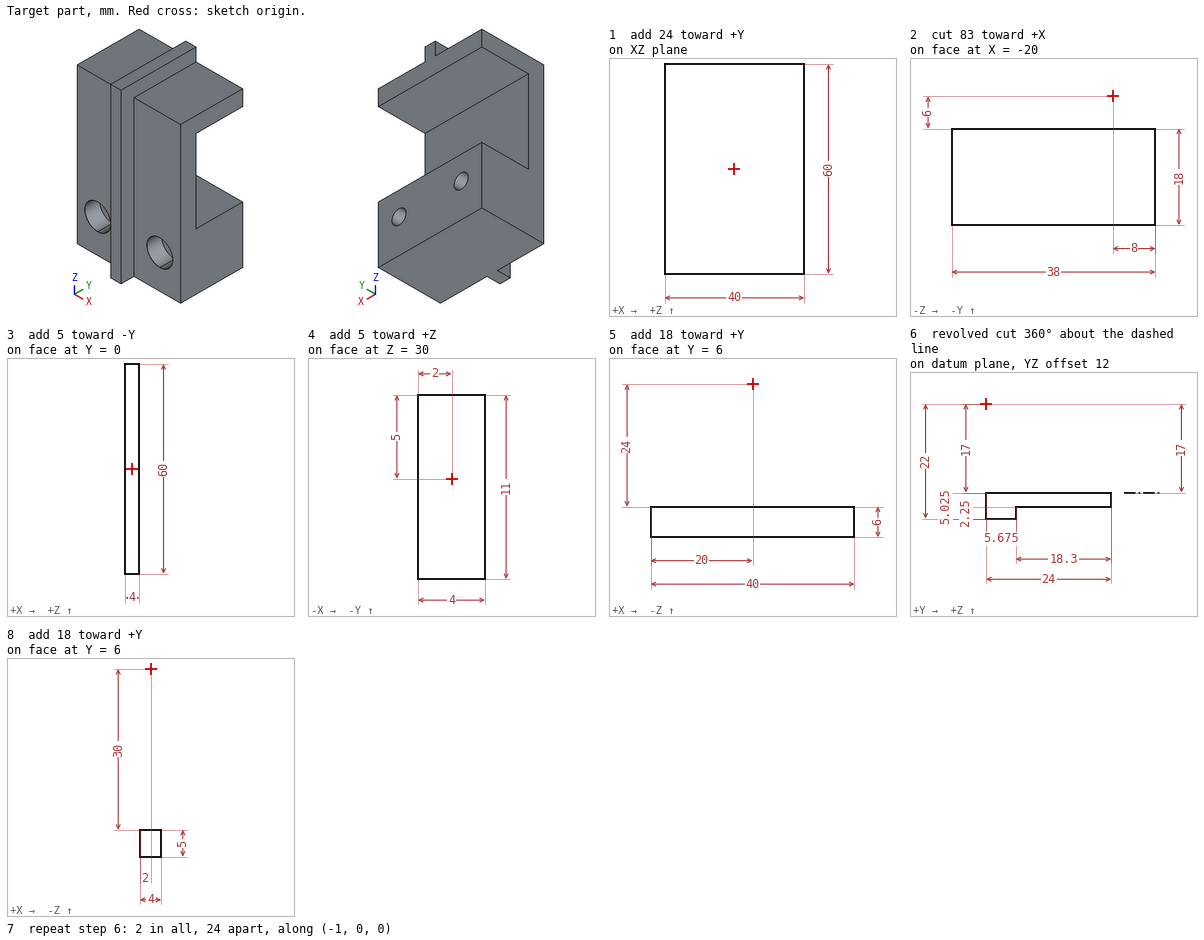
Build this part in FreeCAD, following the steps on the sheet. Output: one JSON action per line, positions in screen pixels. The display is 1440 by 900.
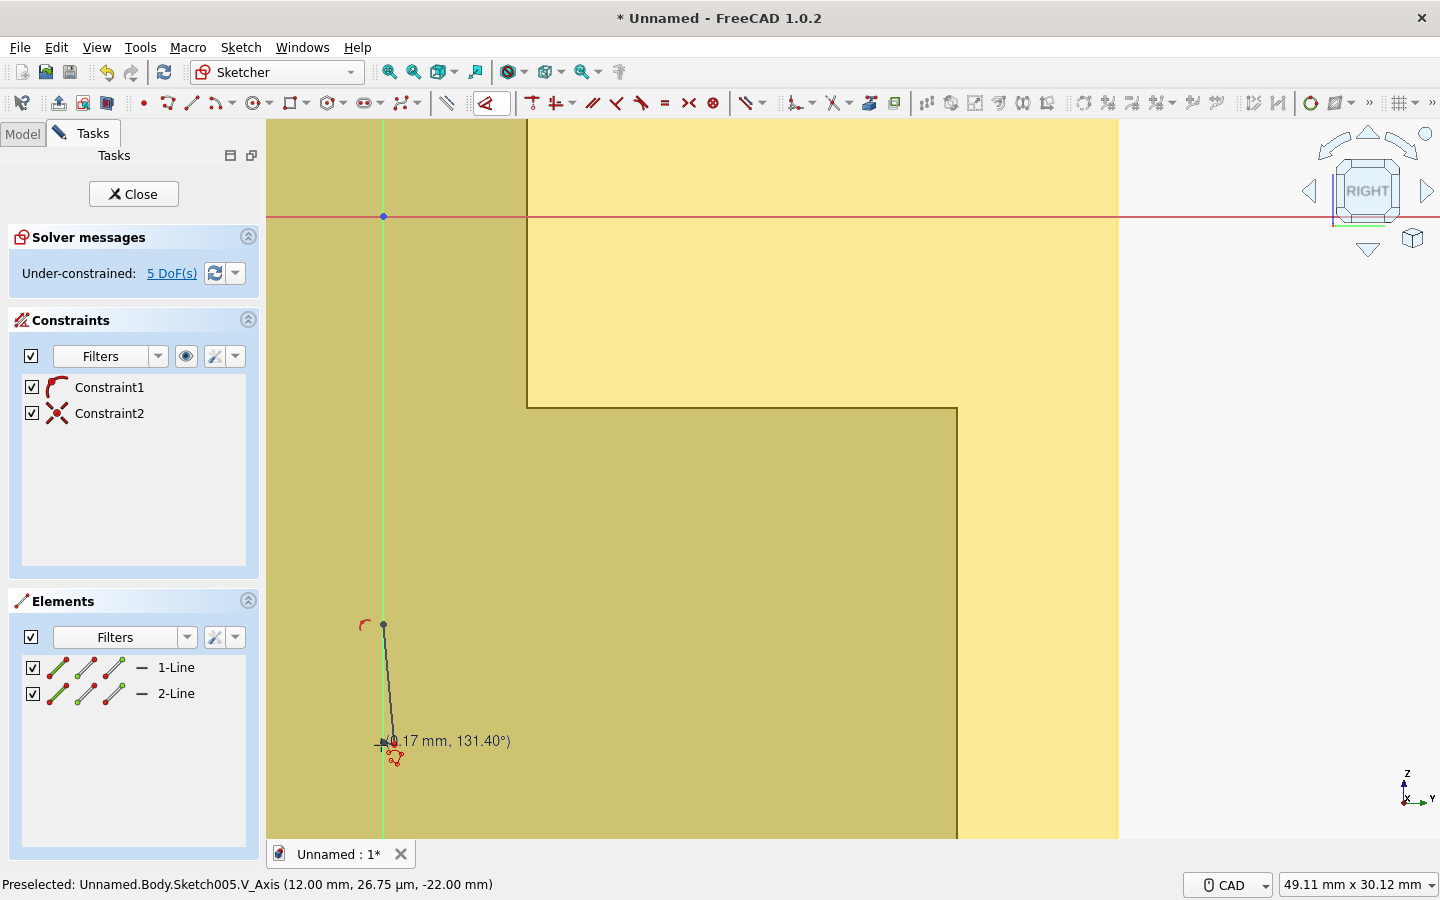
{"action": "left_click", "coordinate": [519, 743]}
{"action": "left_click", "coordinate": [519, 689]}
{"action": "left_click", "coordinate": [957, 689]}
{"action": "left_click", "coordinate": [957, 623]}
{"action": "left_click", "coordinate": [383, 625]}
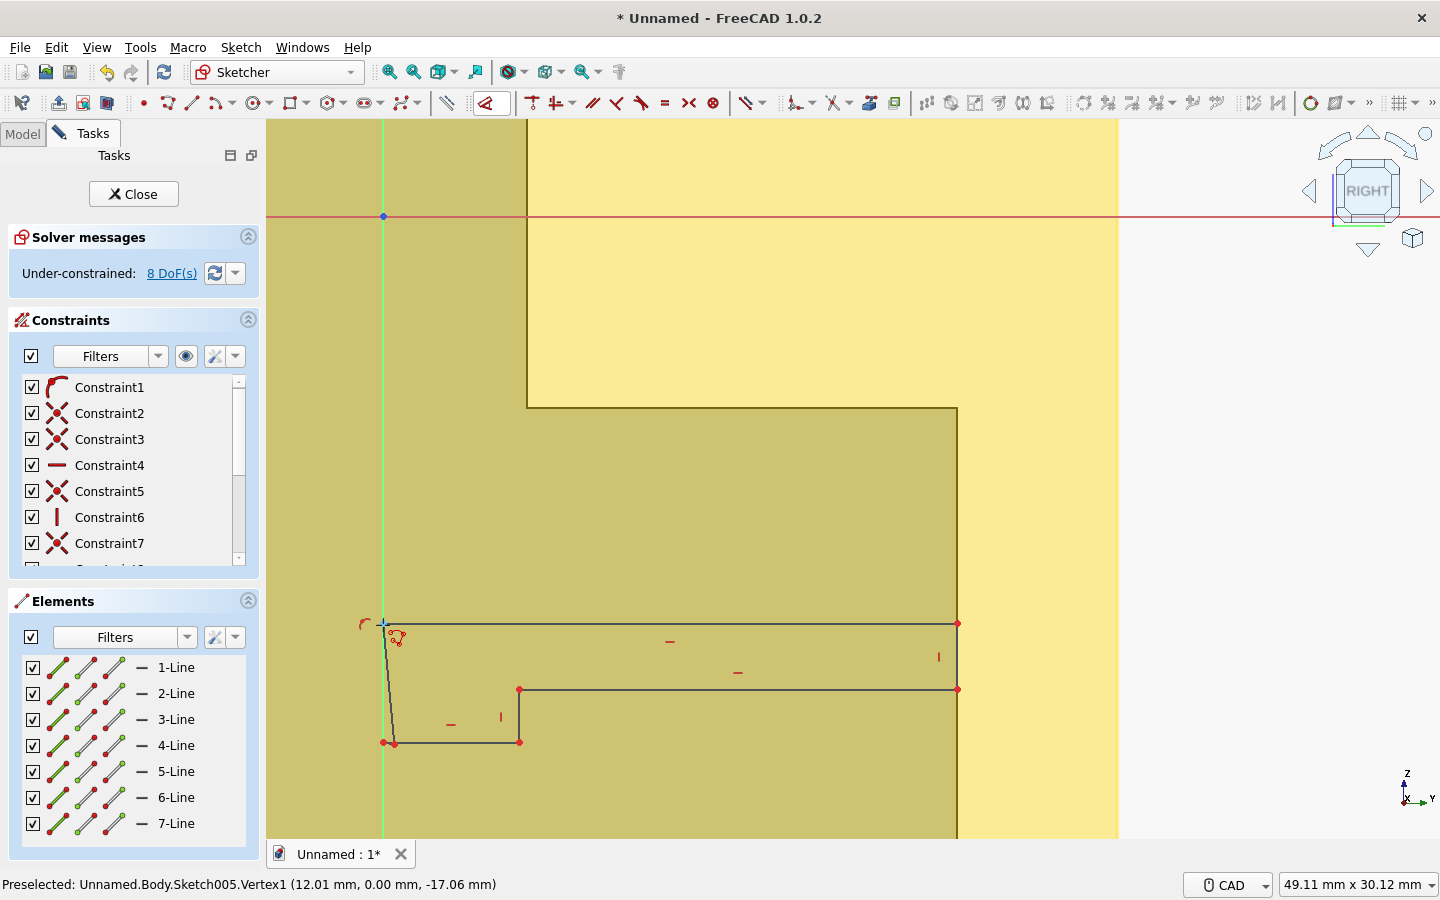
{"action": "key", "text": "g l"}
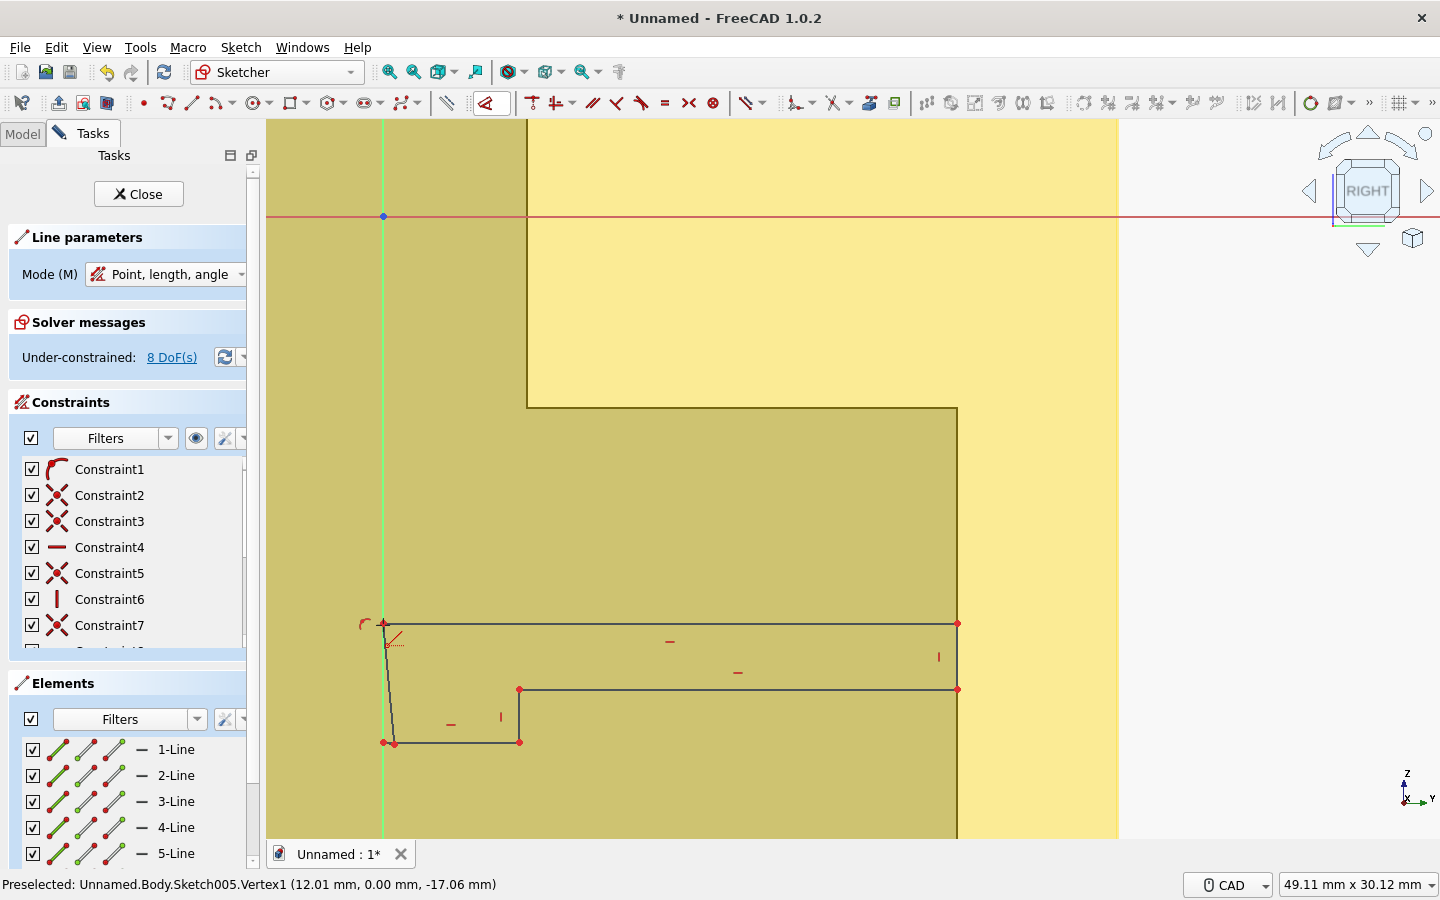
{"action": "left_click", "coordinate": [1014, 623]}
{"action": "left_click", "coordinate": [1186, 623]}
{"action": "key", "text": "Escape"}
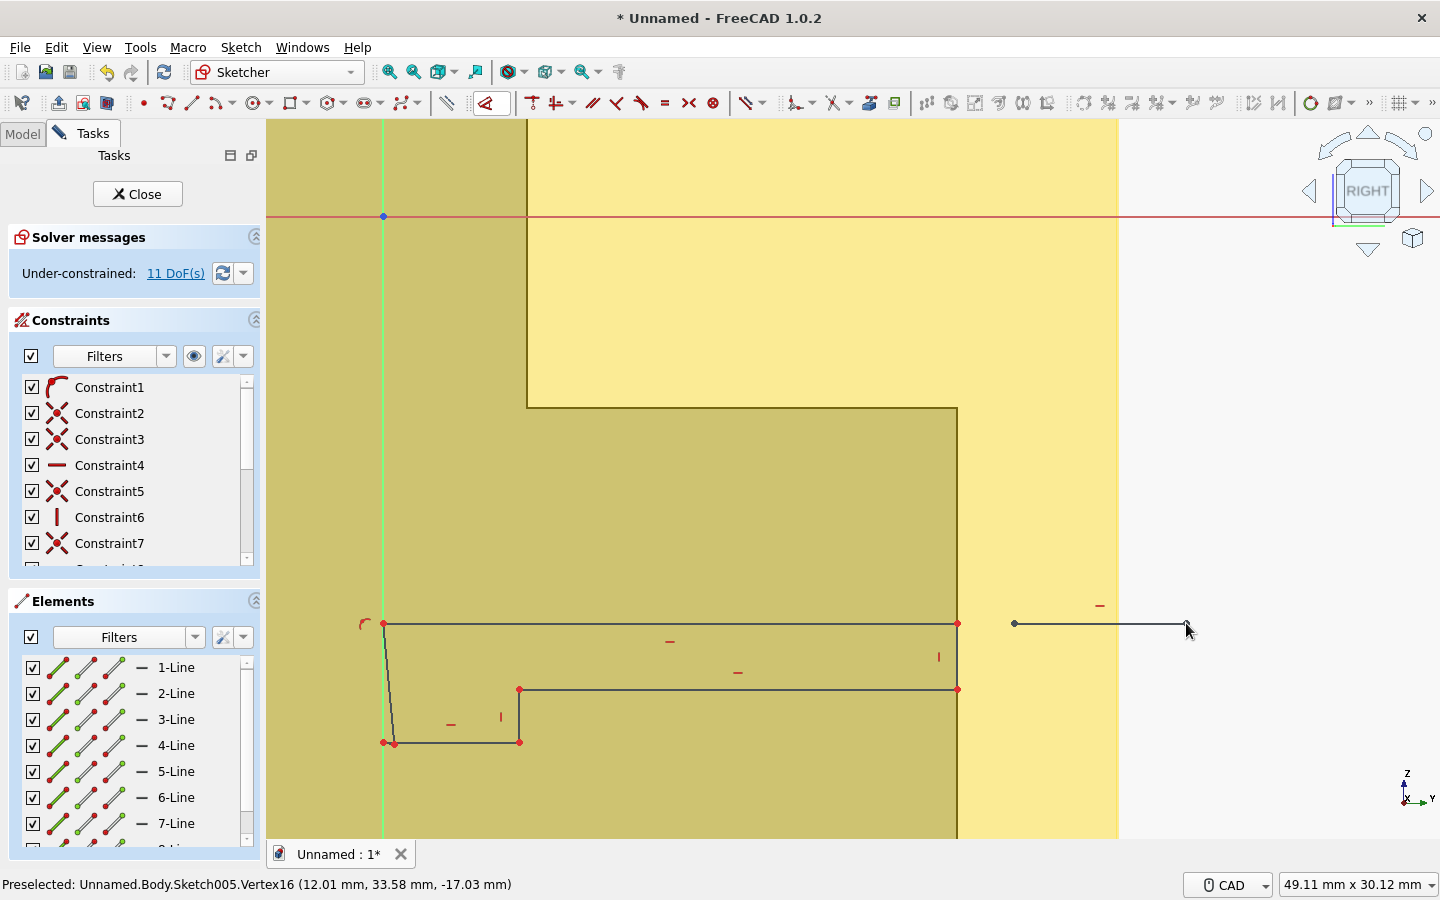
{"action": "left_click", "coordinate": [1066, 624]}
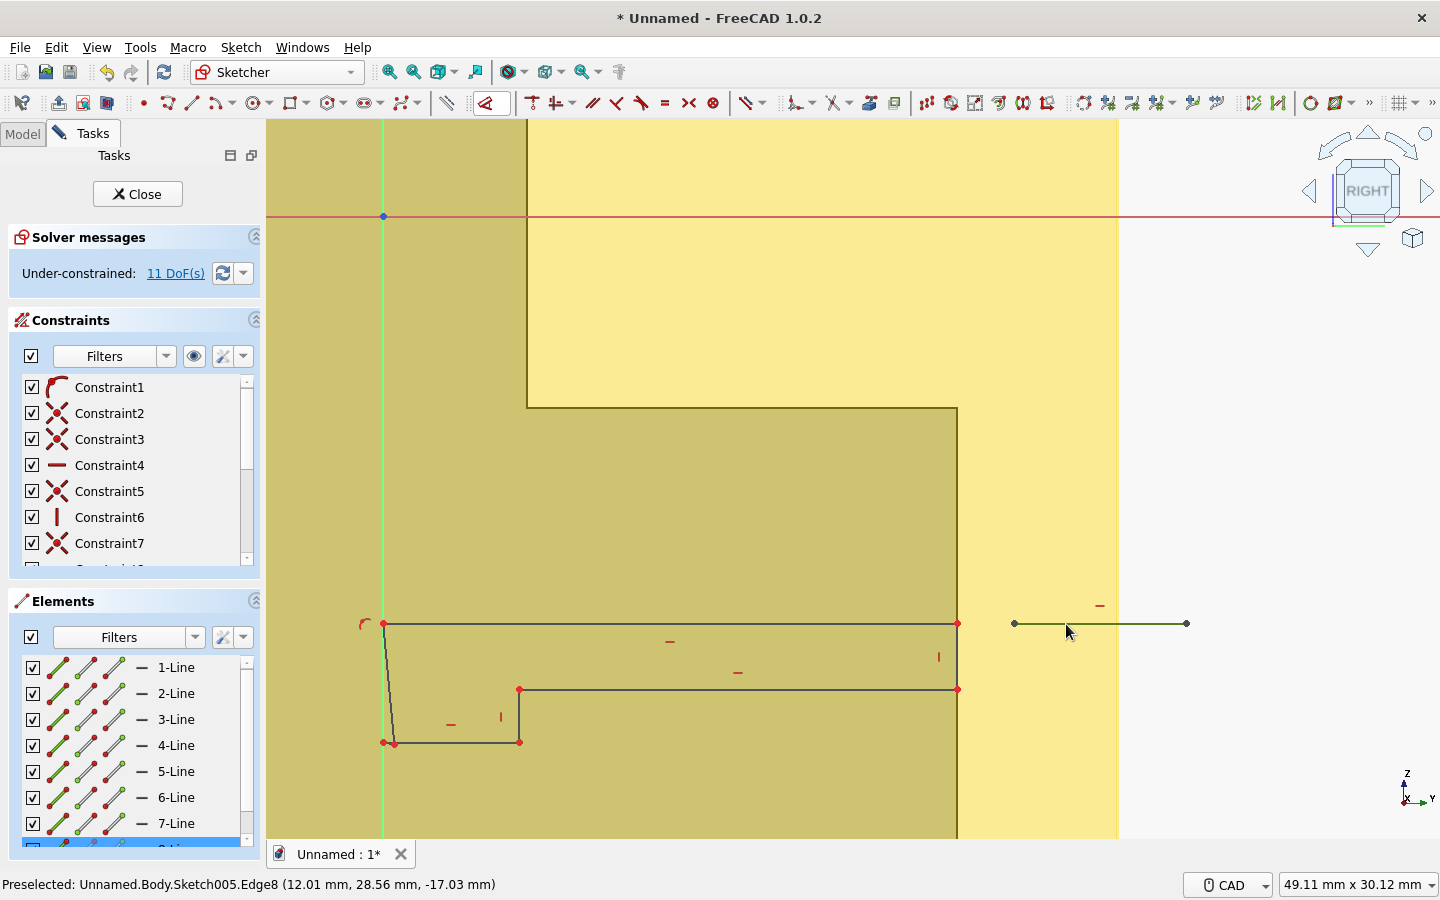
{"action": "key", "text": "g n"}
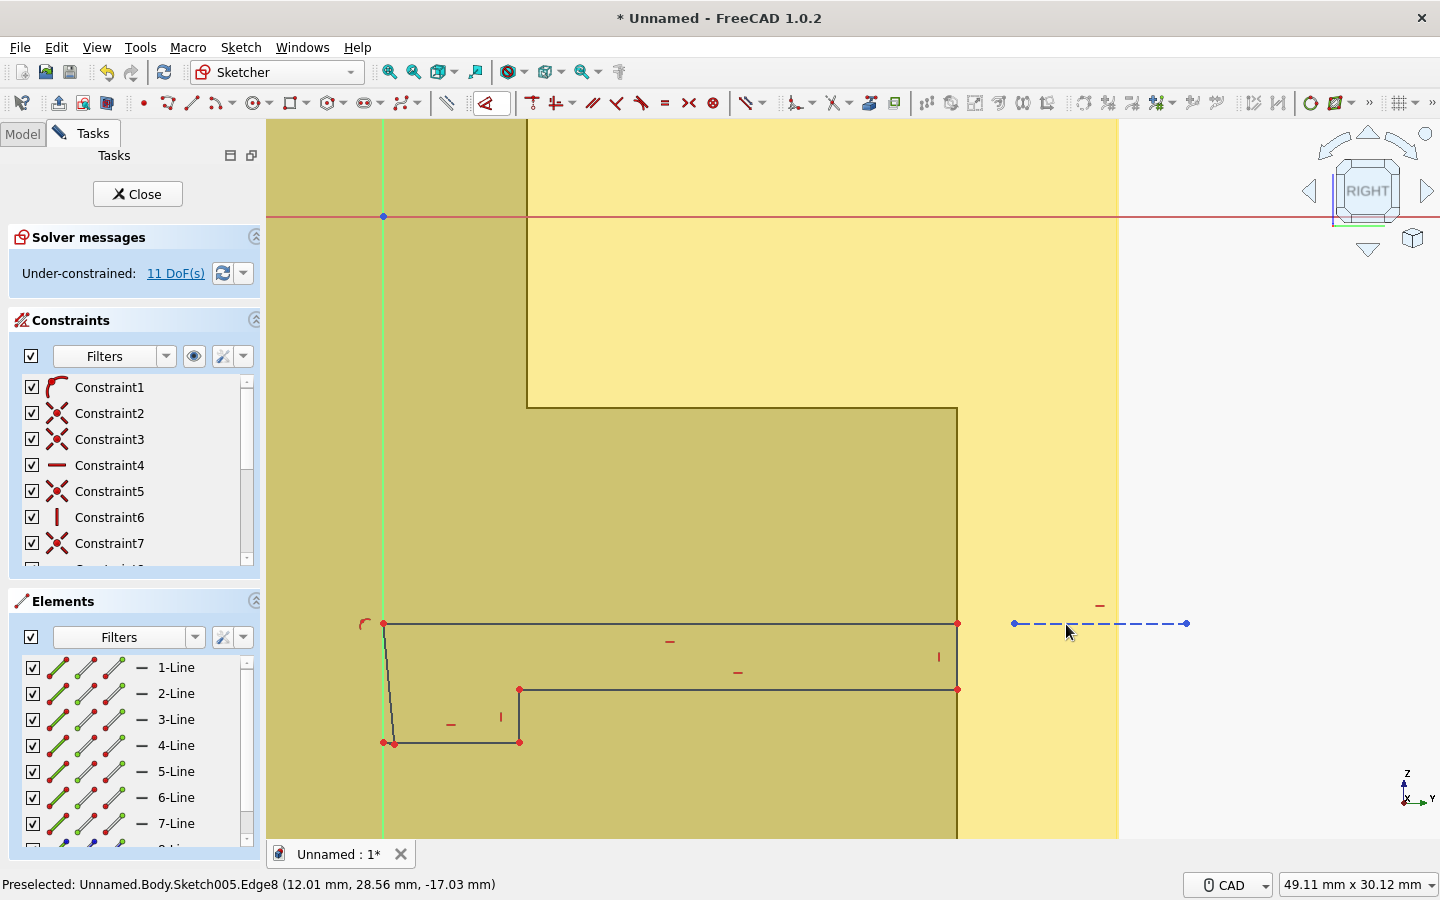
{"action": "left_click", "coordinate": [387, 660]}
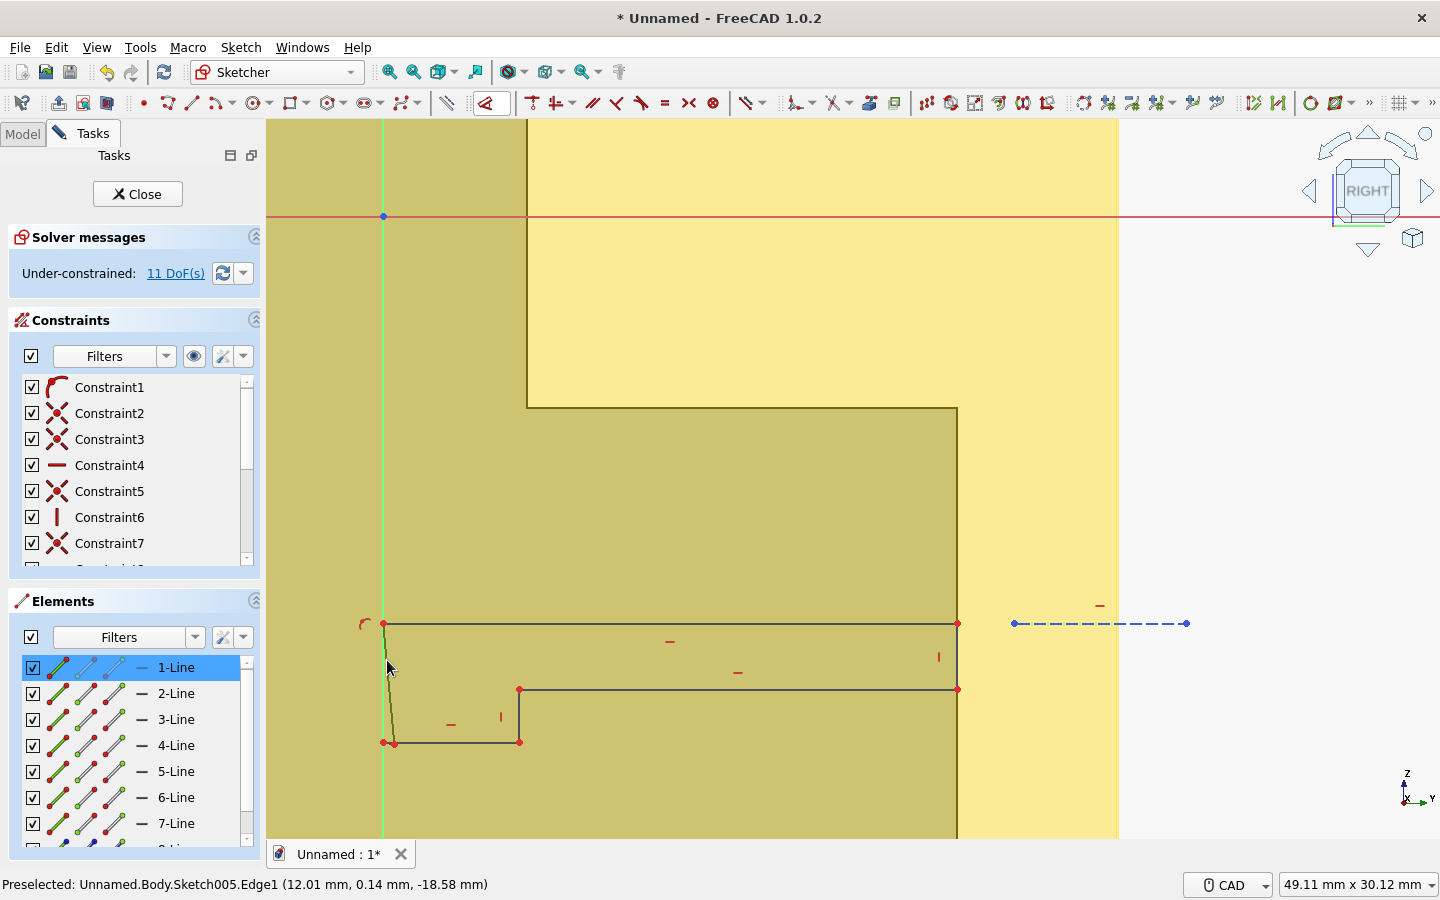
{"action": "key", "text": "v"}